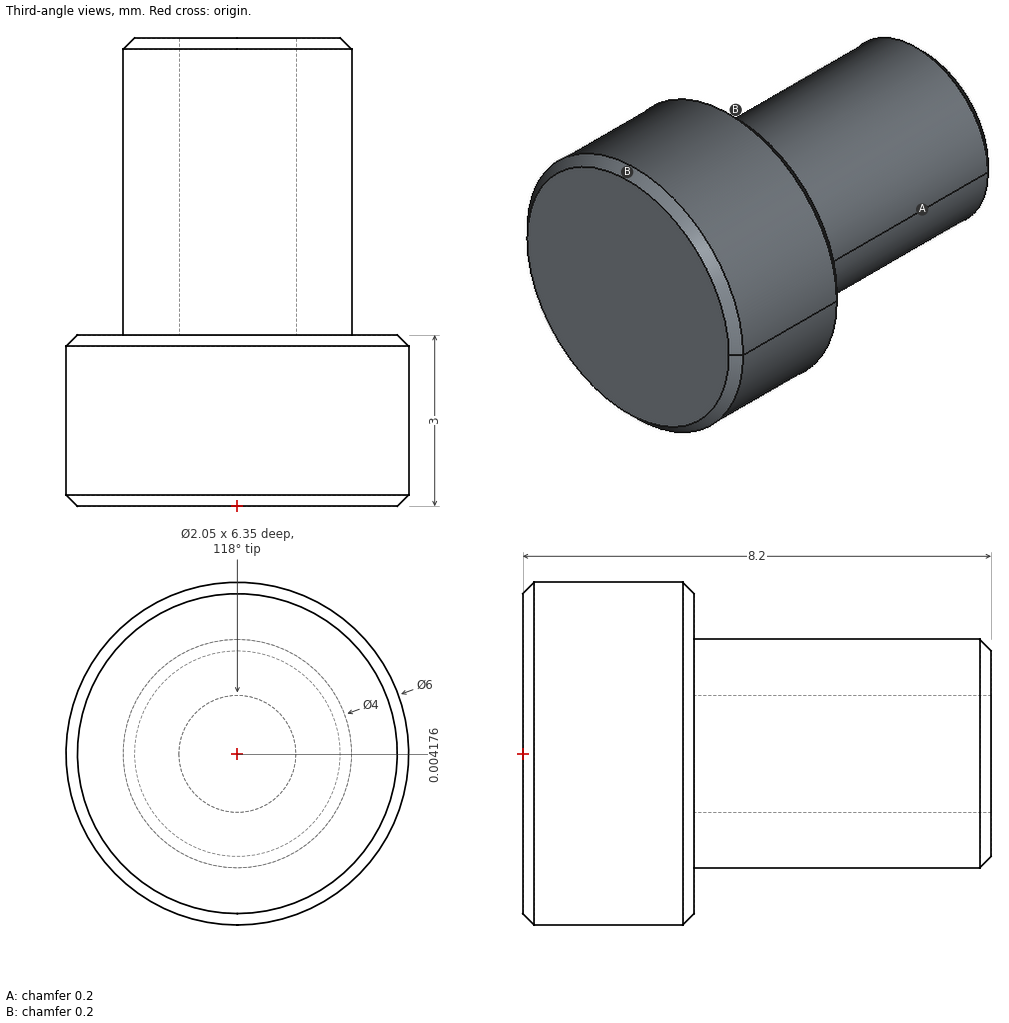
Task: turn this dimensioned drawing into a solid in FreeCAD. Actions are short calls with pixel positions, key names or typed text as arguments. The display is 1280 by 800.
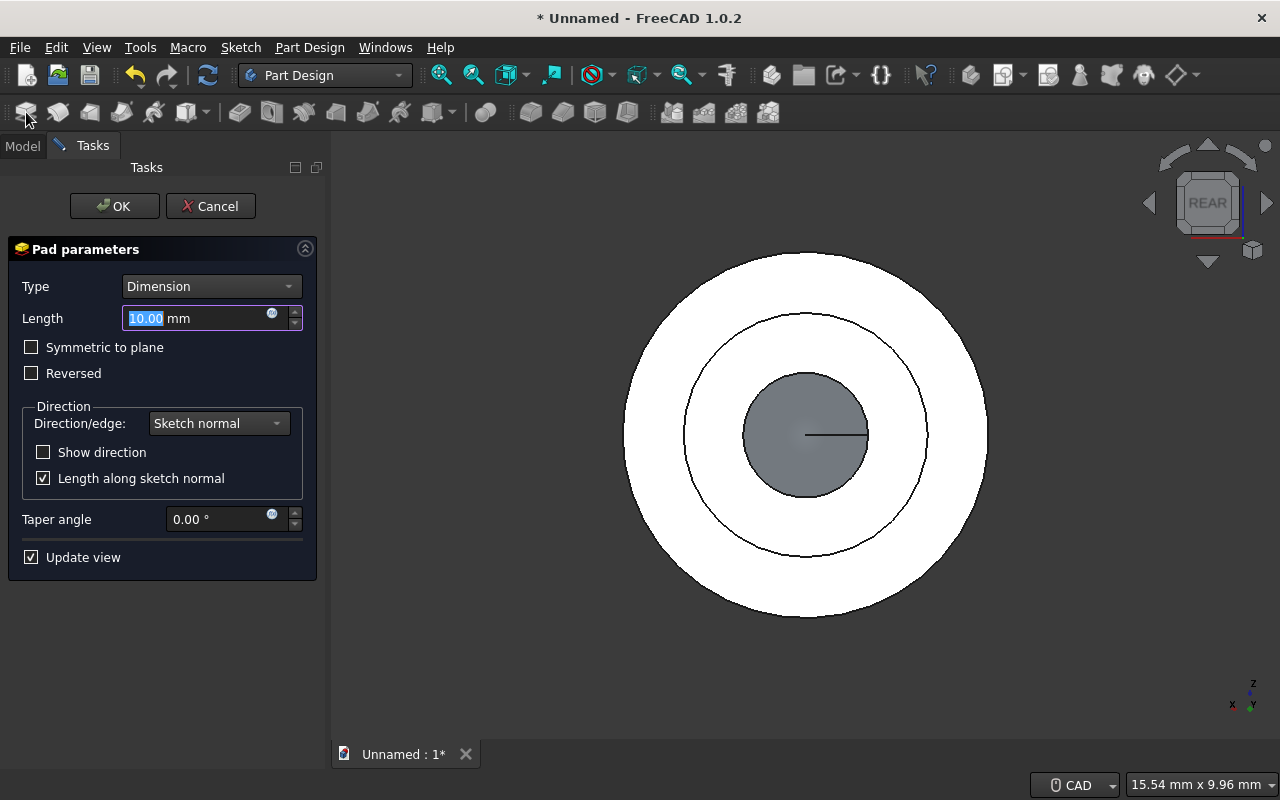
text(3)
key(Tab)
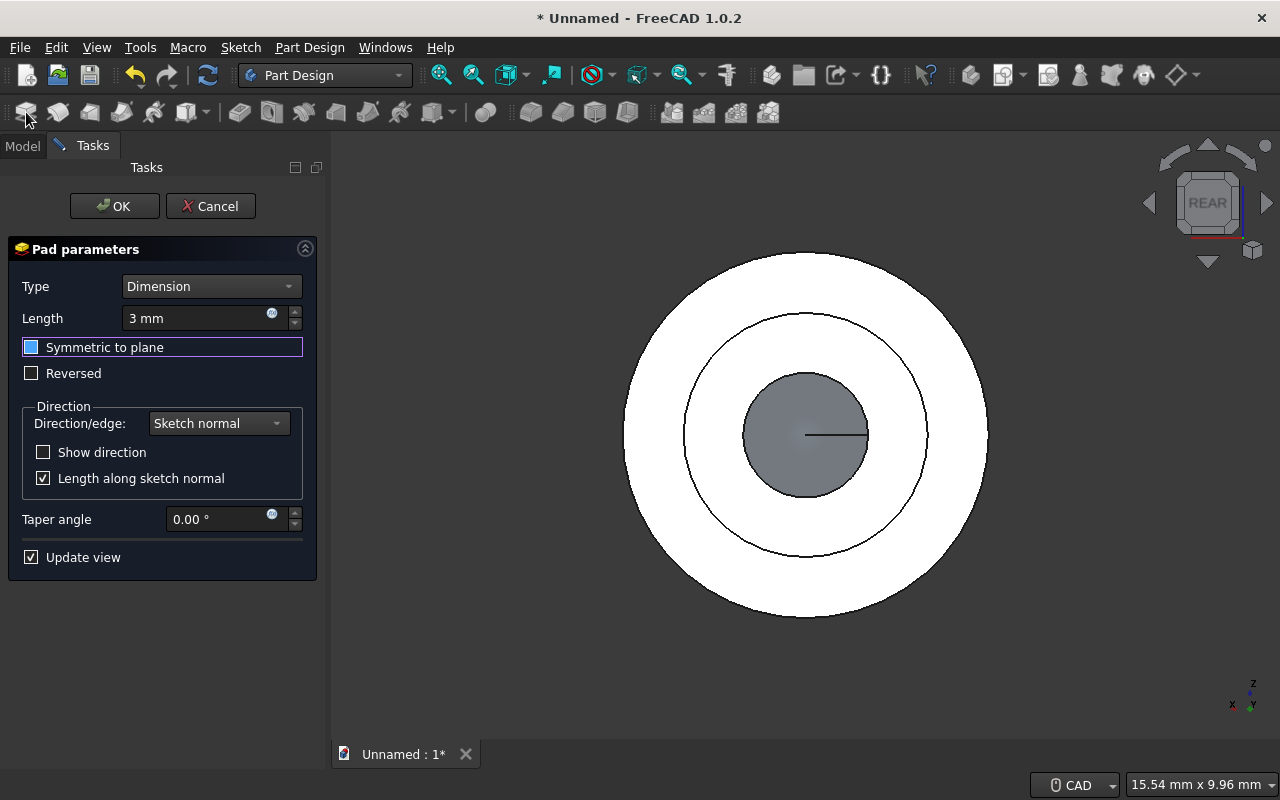
click(30, 373)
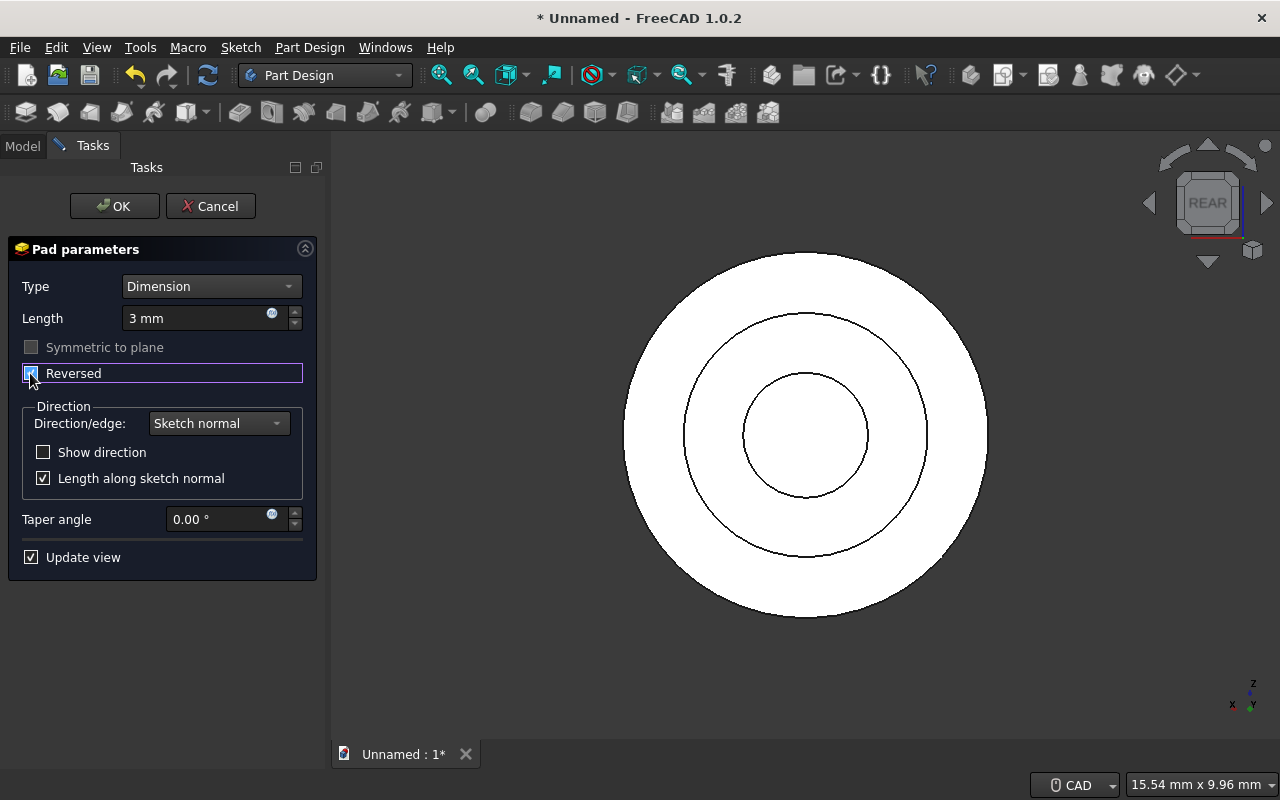
click(115, 206)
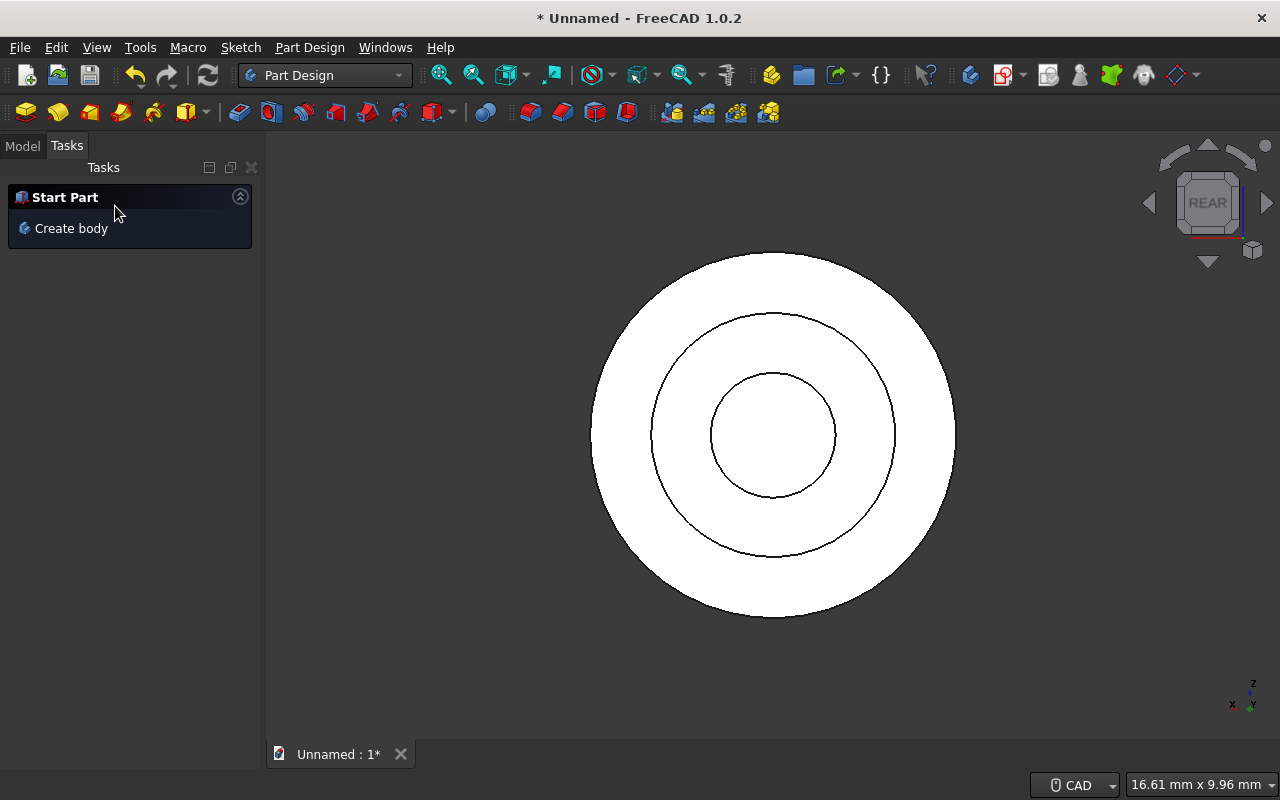
click(895, 434)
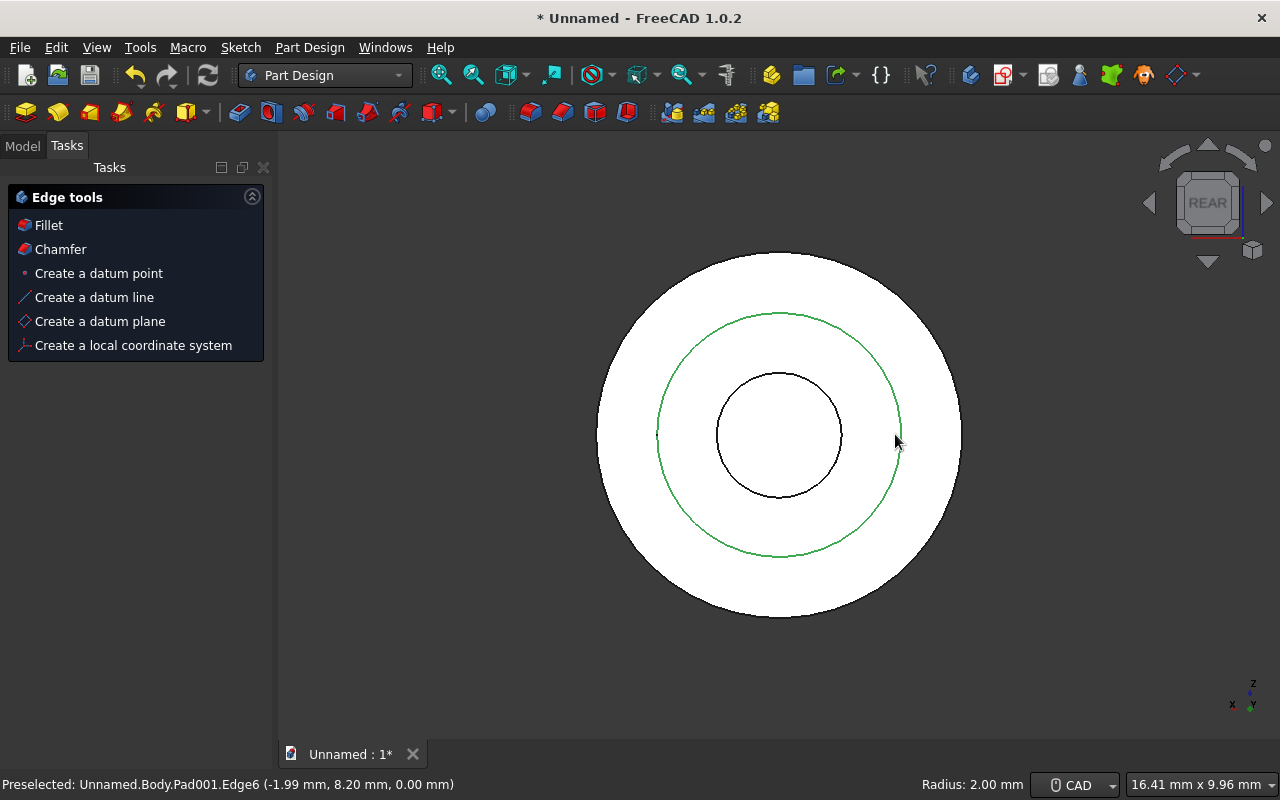
click(564, 112)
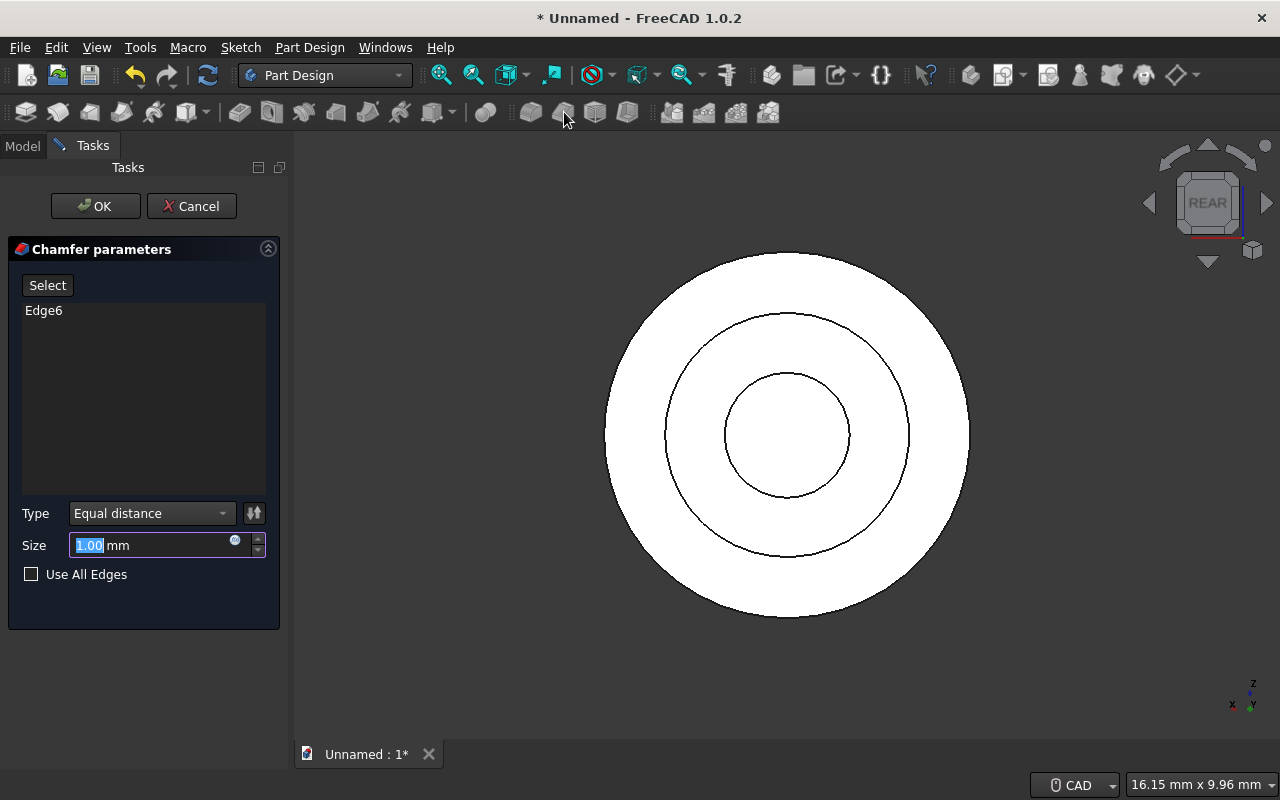
text(0.2)
key(Tab)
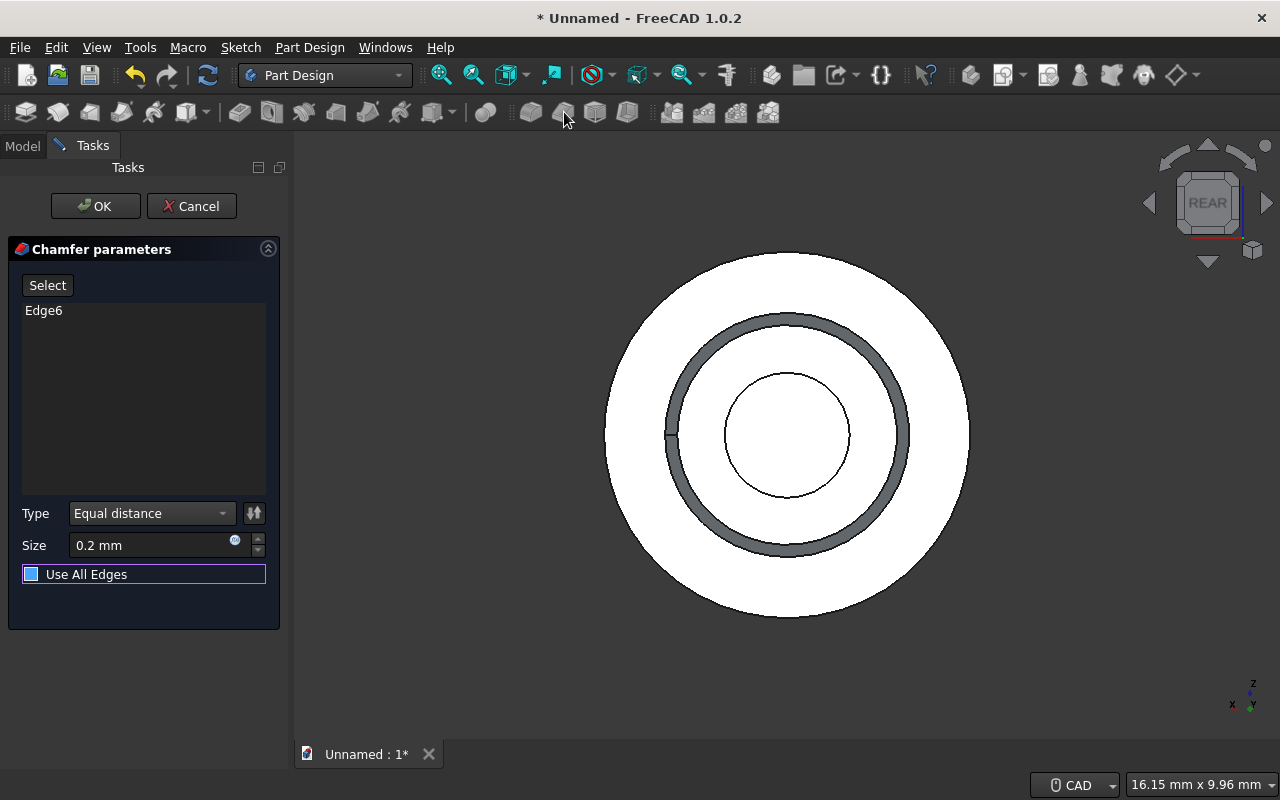
click(96, 206)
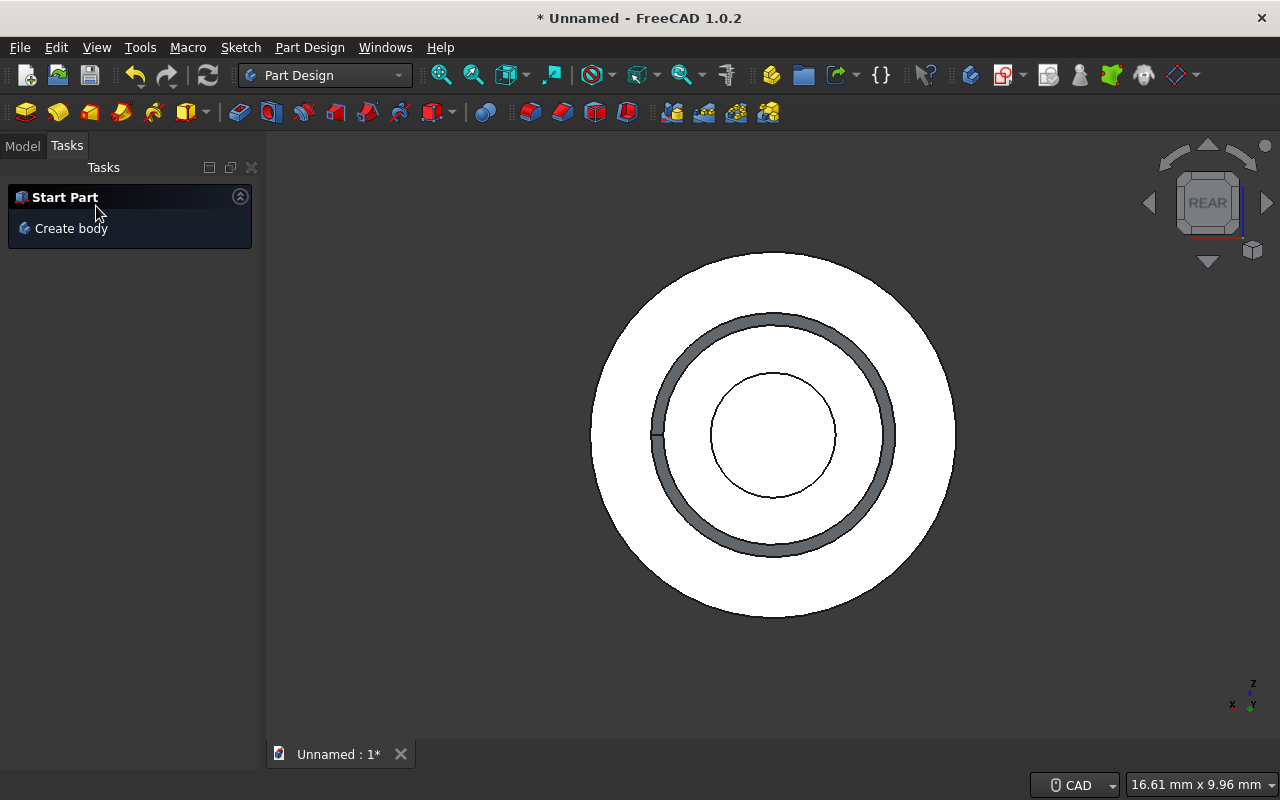
click(956, 434)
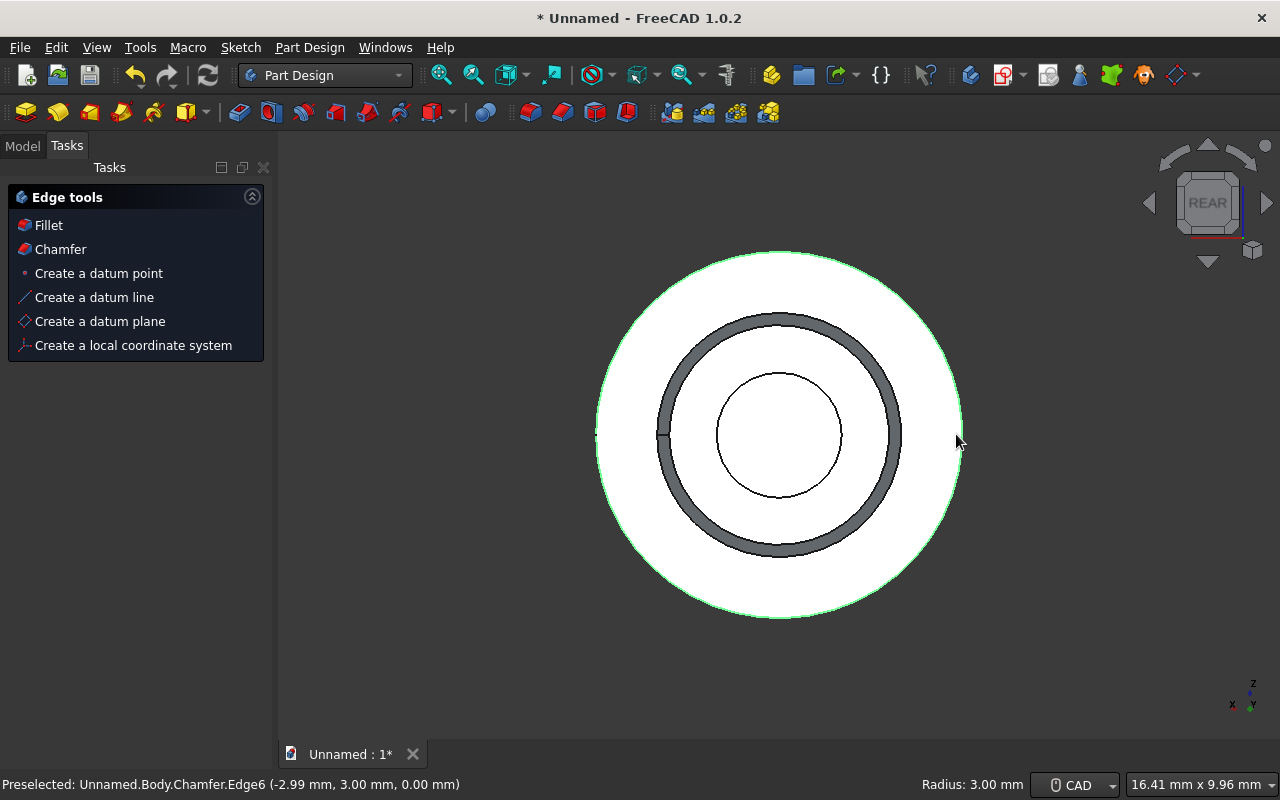
key(0)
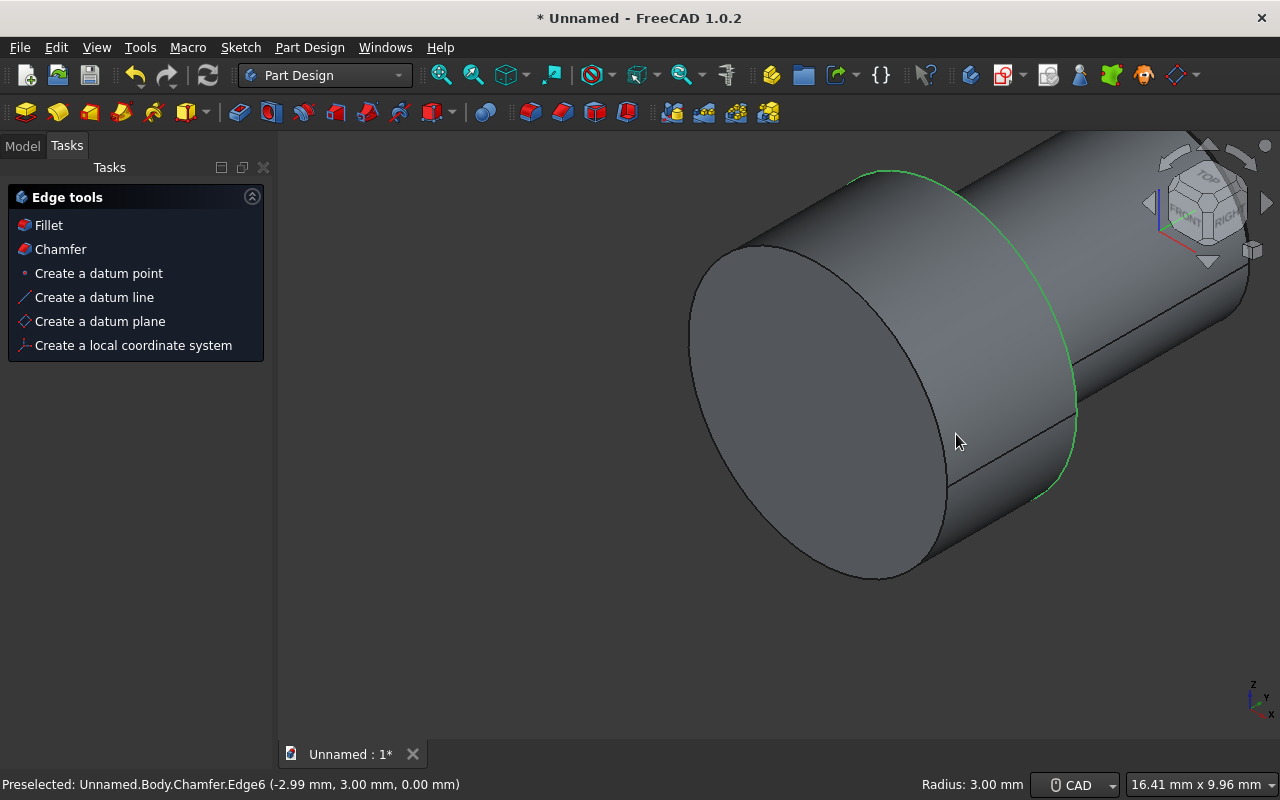
click(442, 76)